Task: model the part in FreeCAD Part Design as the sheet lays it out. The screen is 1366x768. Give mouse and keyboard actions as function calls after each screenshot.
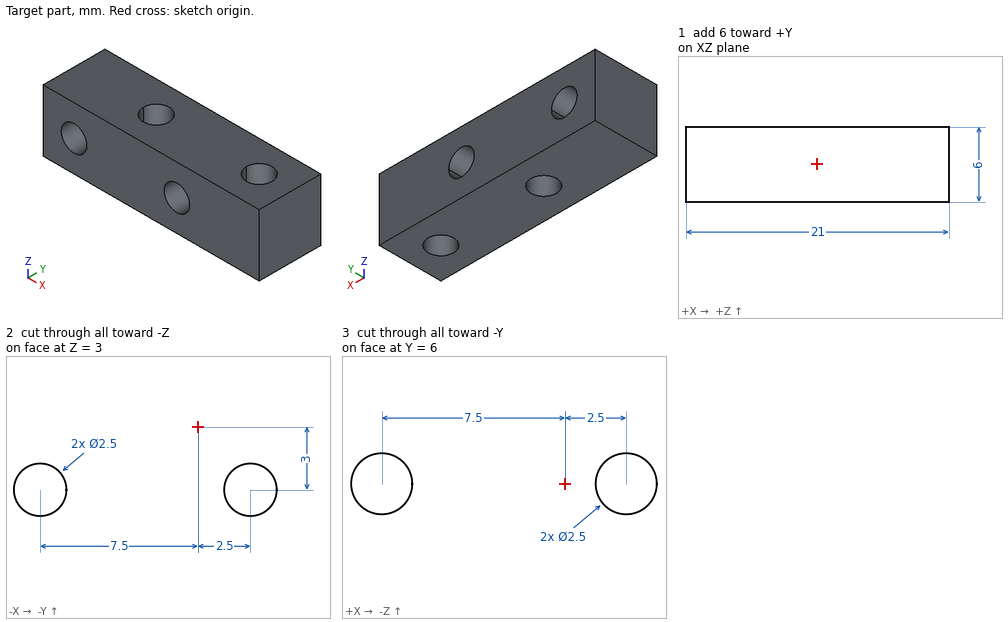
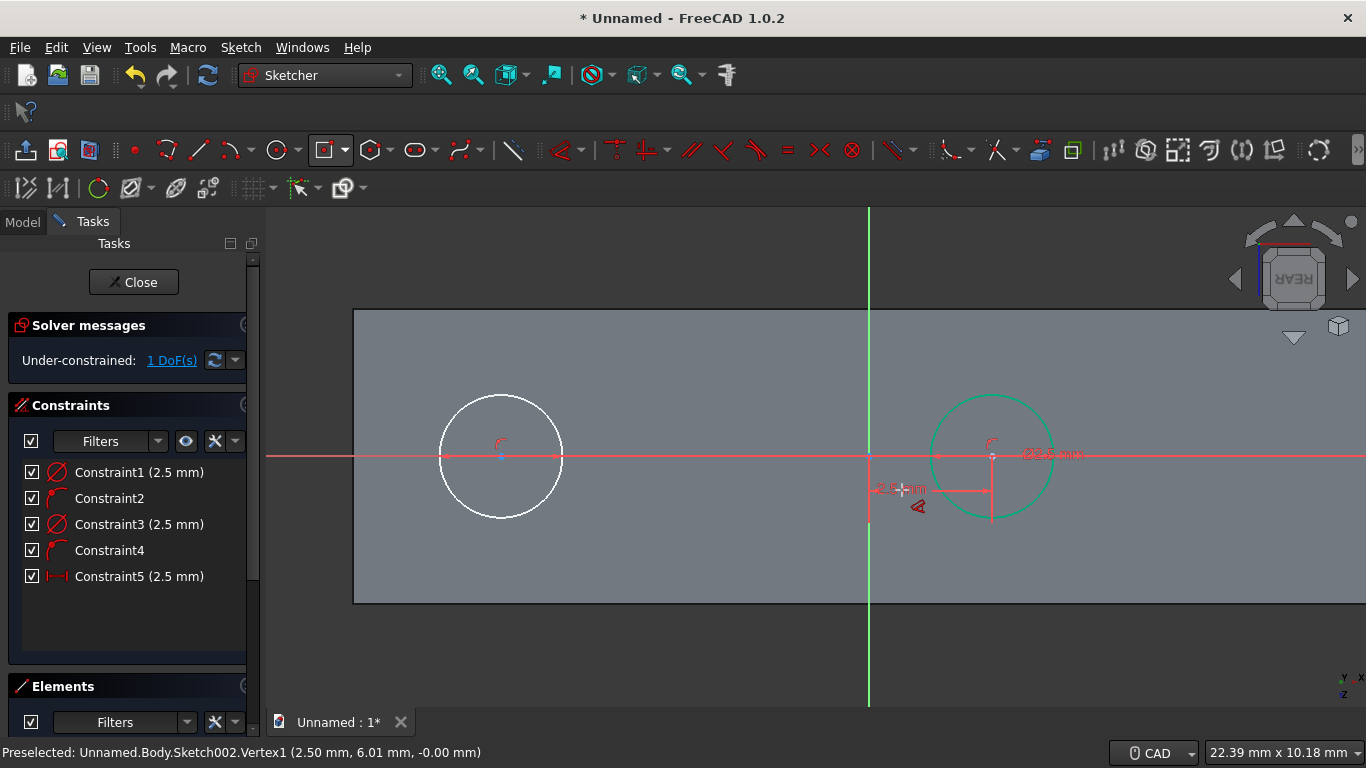
click(501, 456)
click(685, 490)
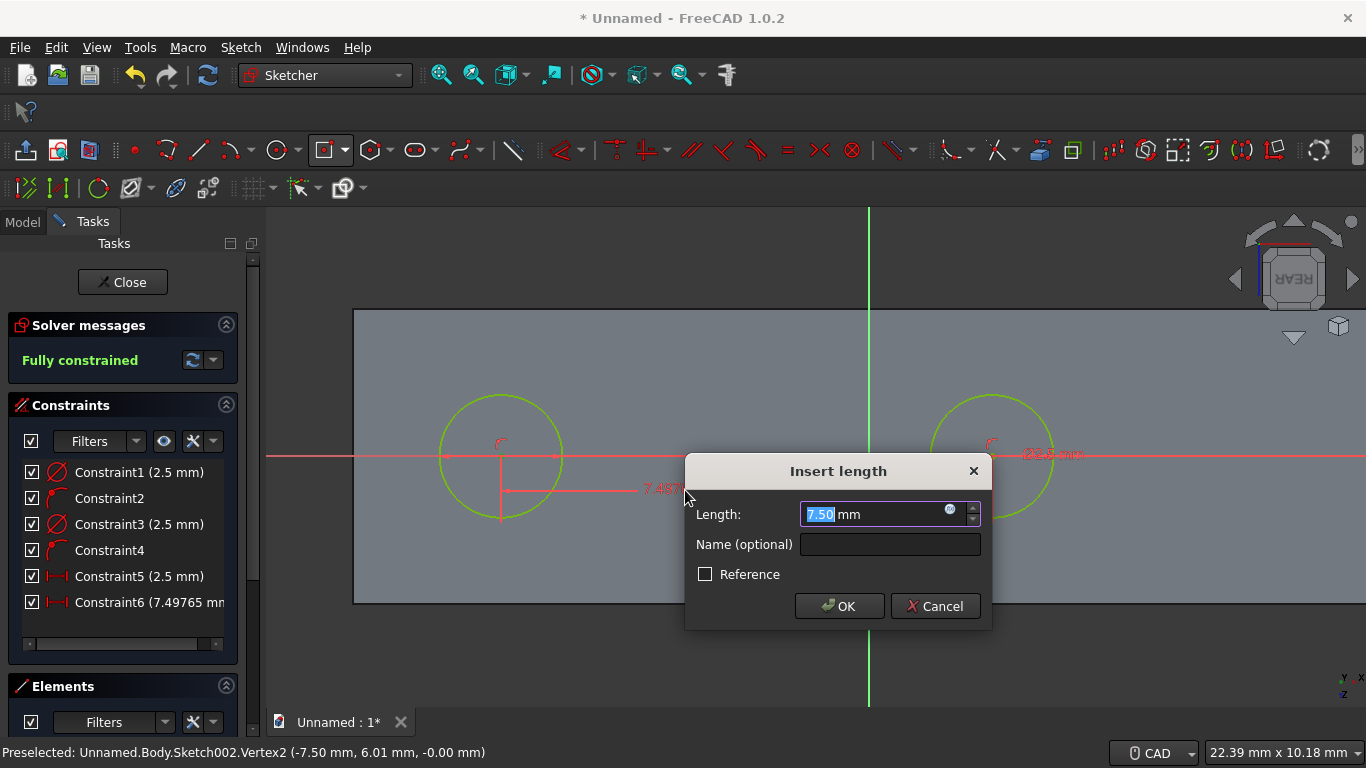
text(7.5)
key(Return)
key(Escape)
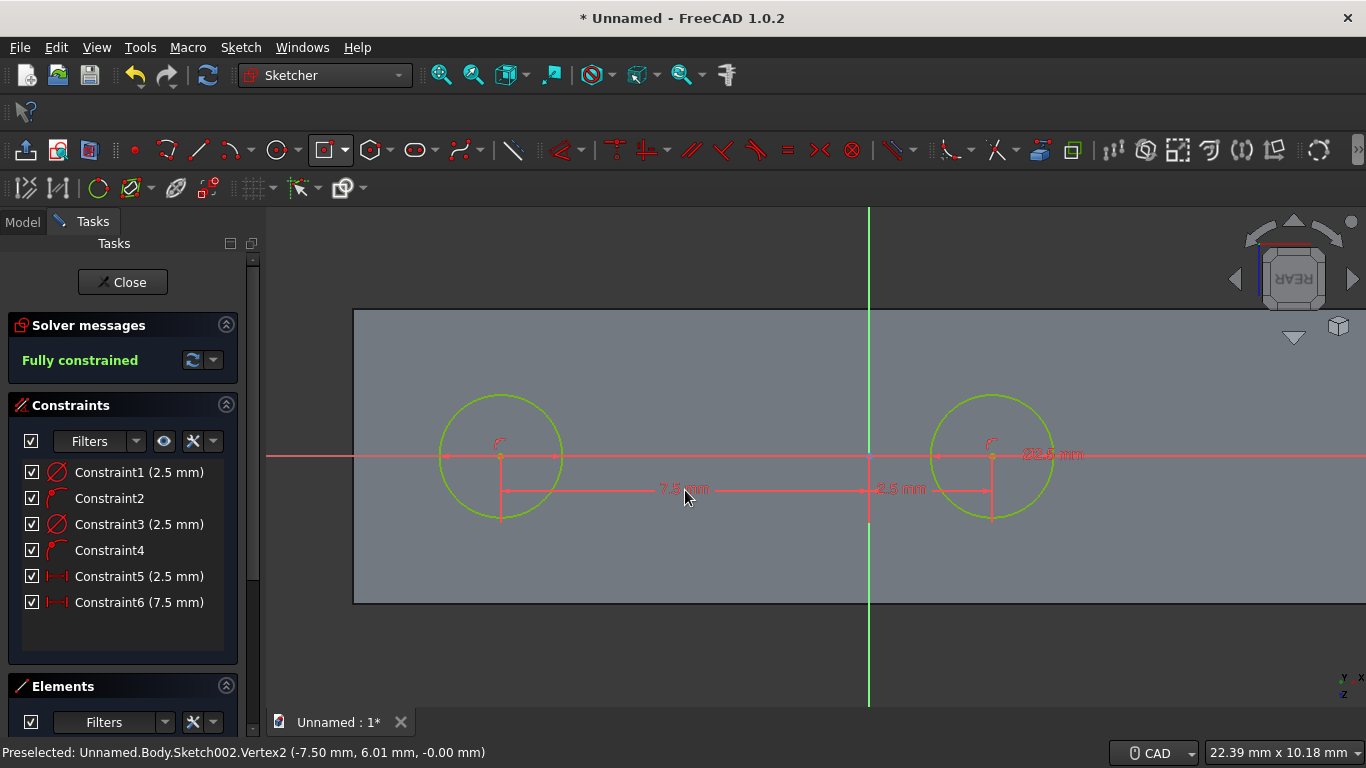
click(123, 282)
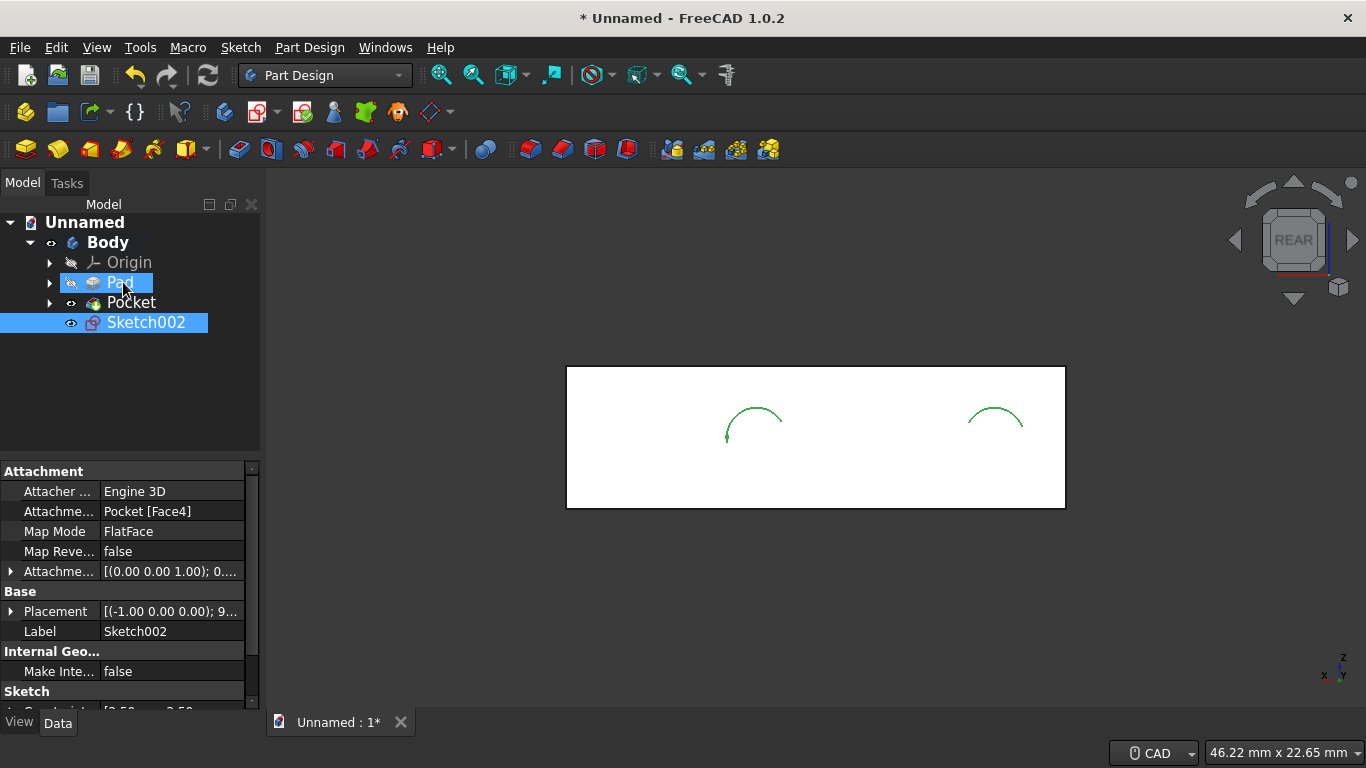
click(240, 150)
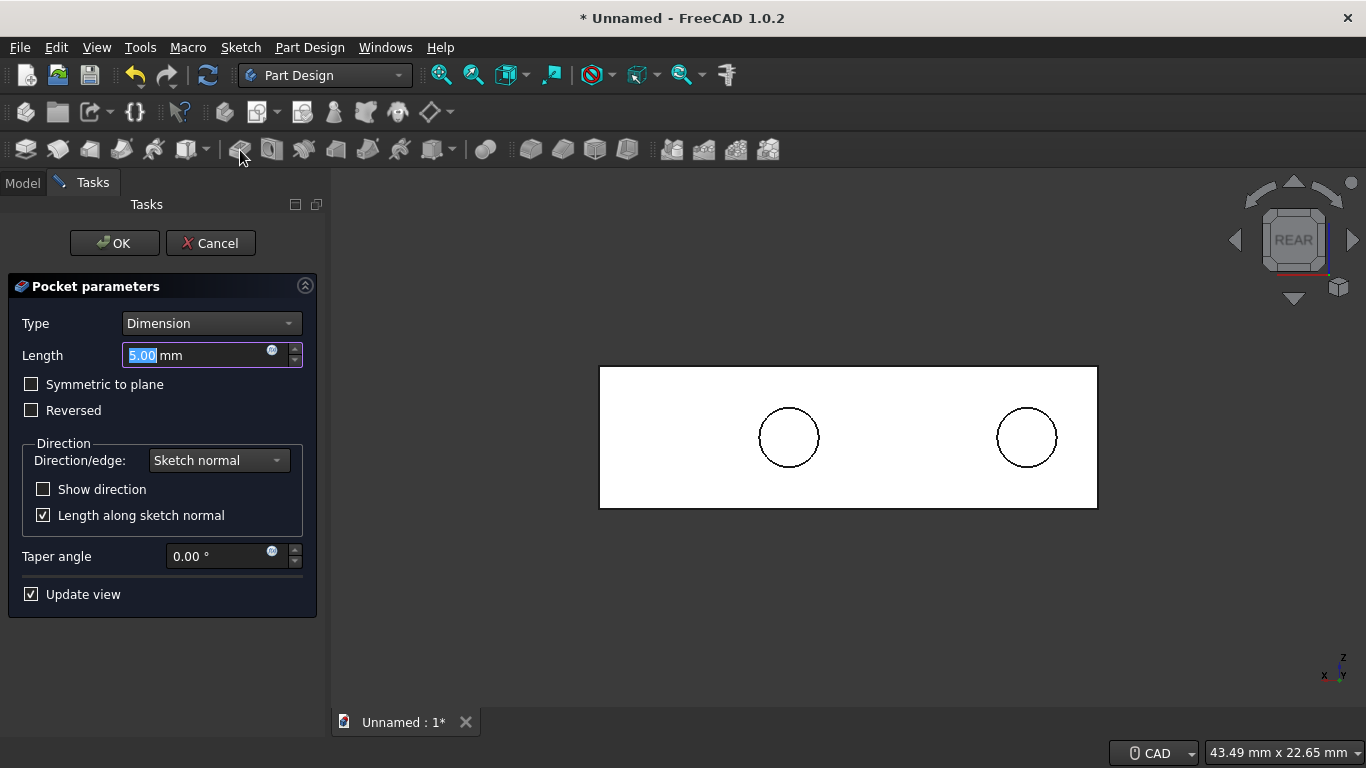
click(212, 324)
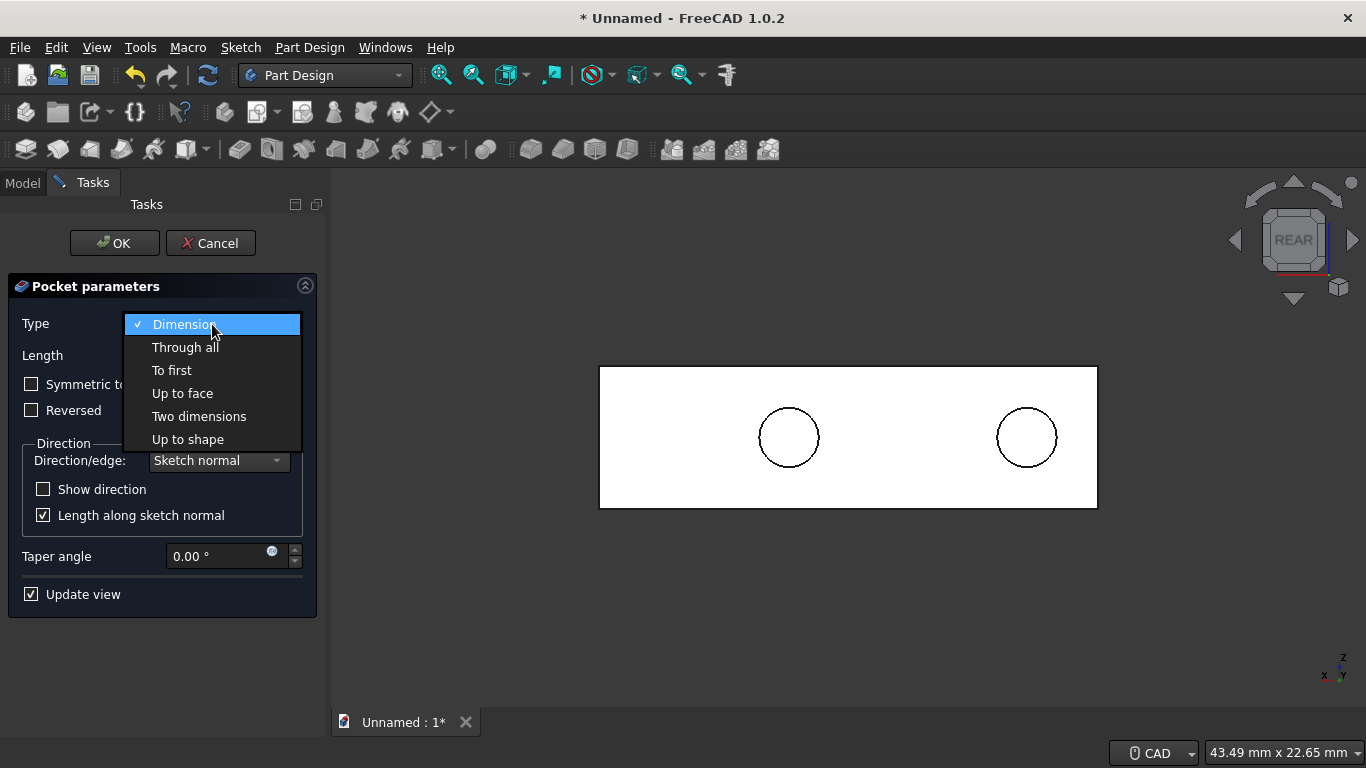
click(212, 348)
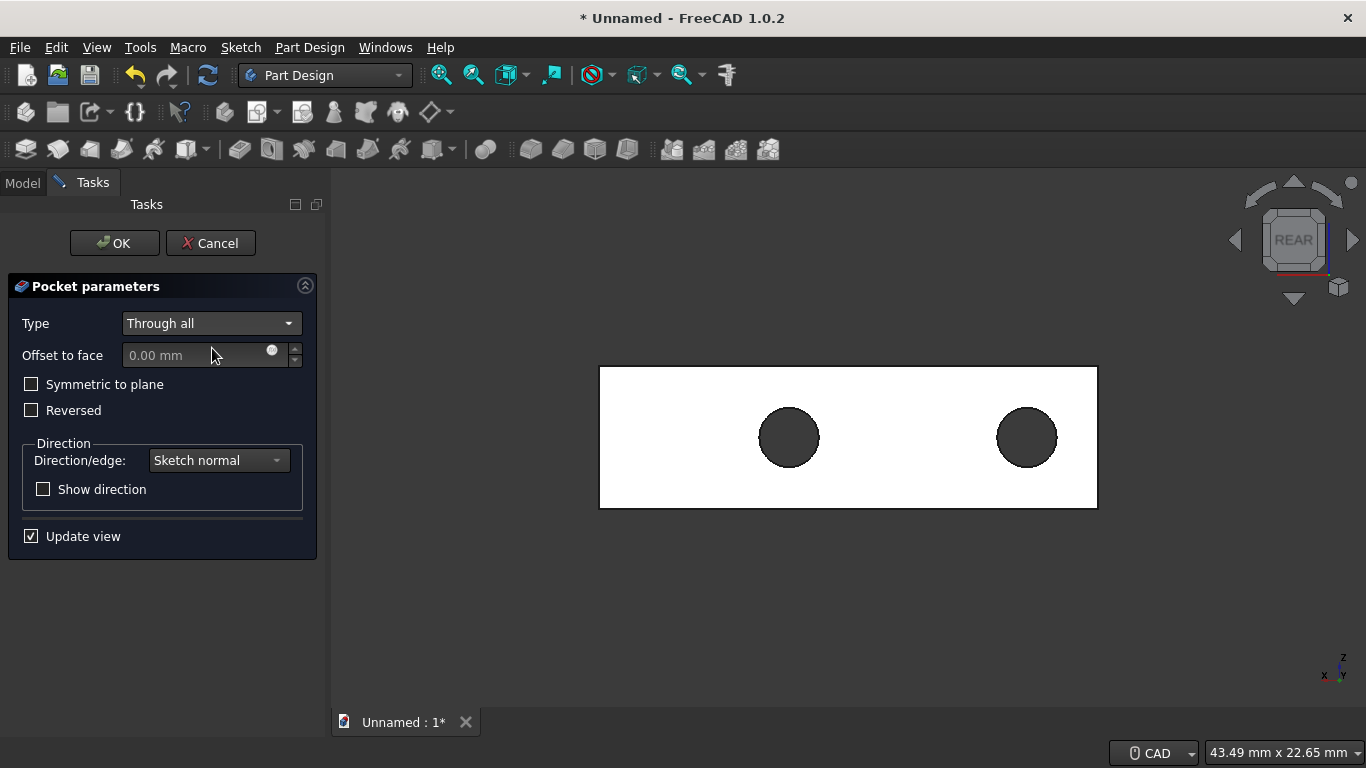
click(115, 243)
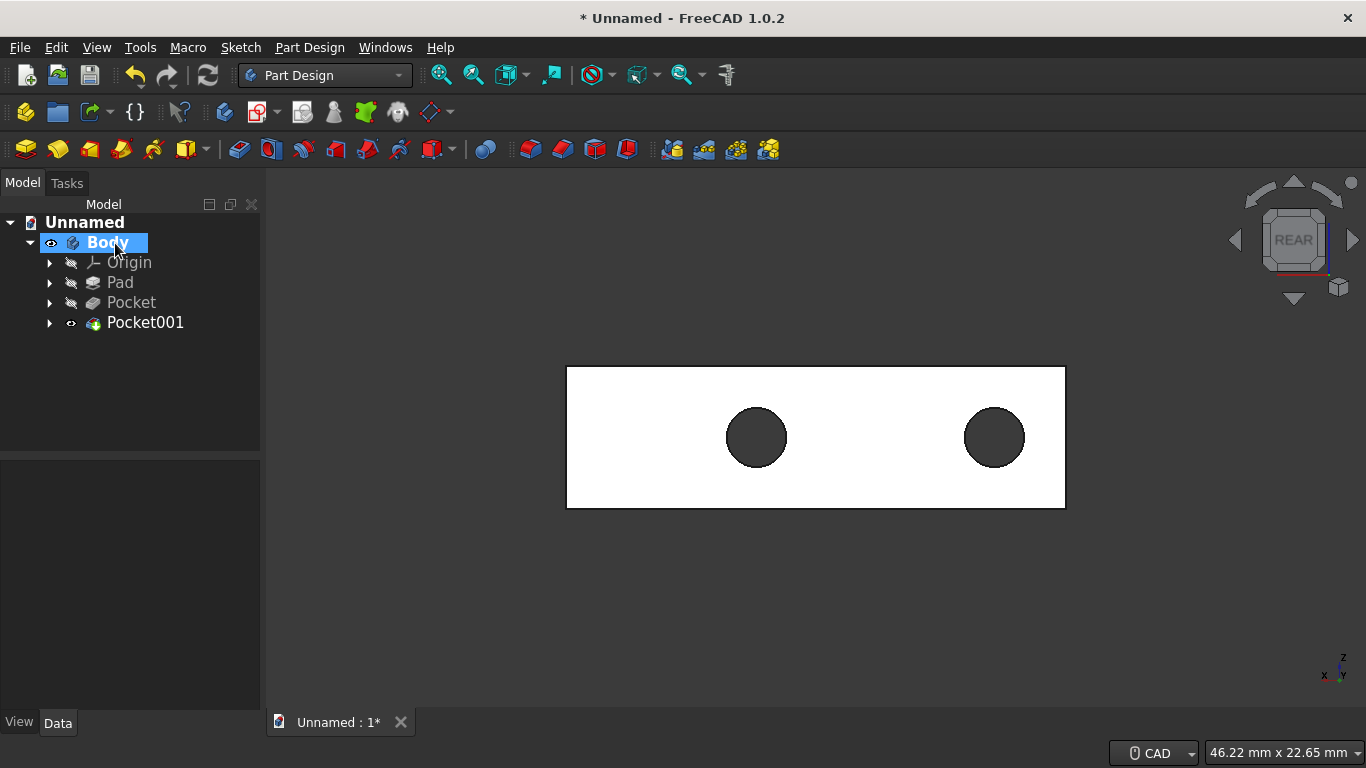
key(0)